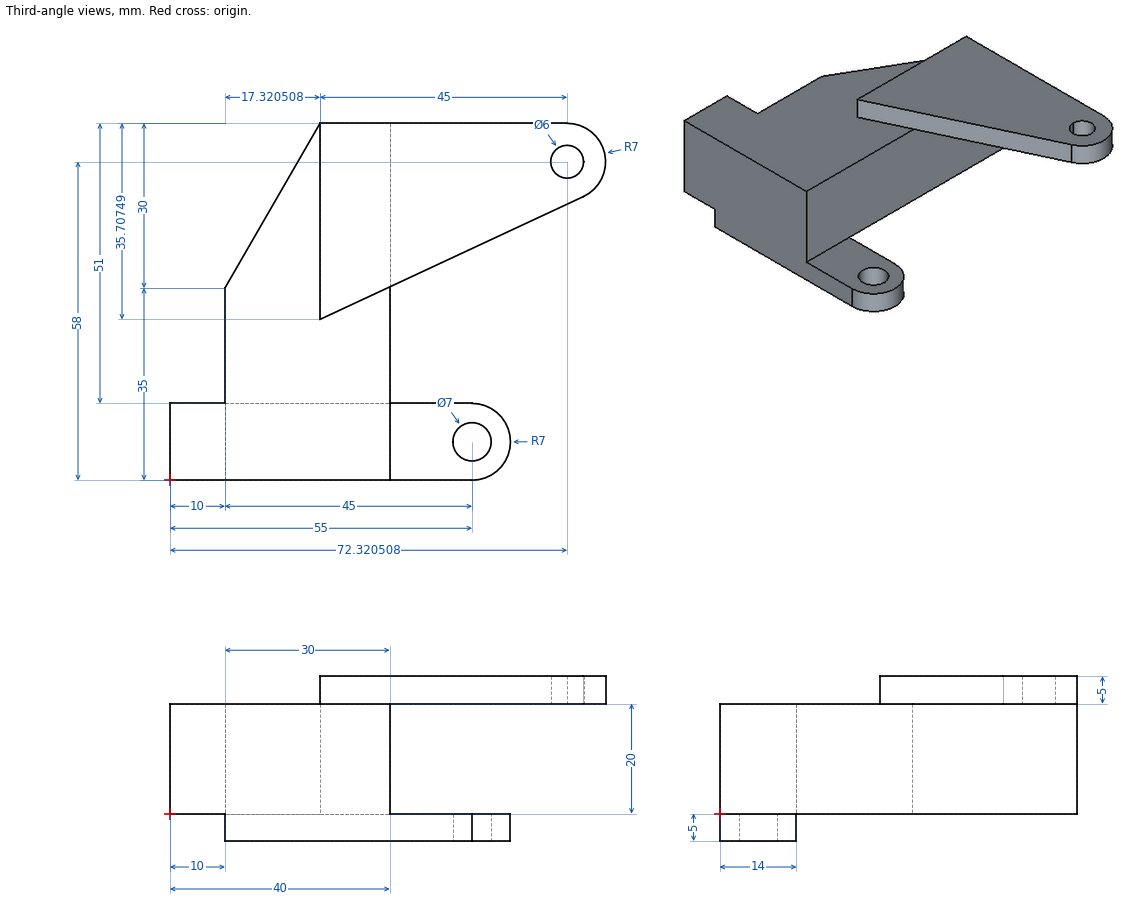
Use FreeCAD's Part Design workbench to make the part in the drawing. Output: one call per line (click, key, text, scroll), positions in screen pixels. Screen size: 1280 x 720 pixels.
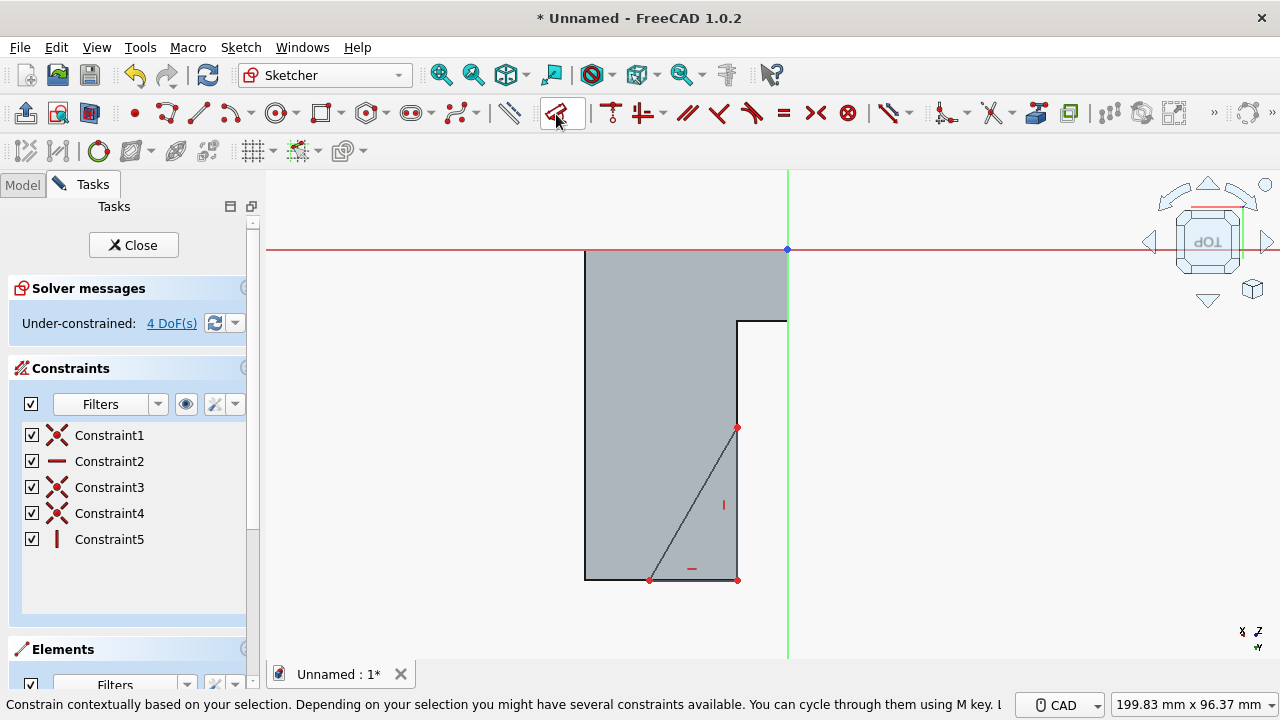
click(737, 535)
click(771, 505)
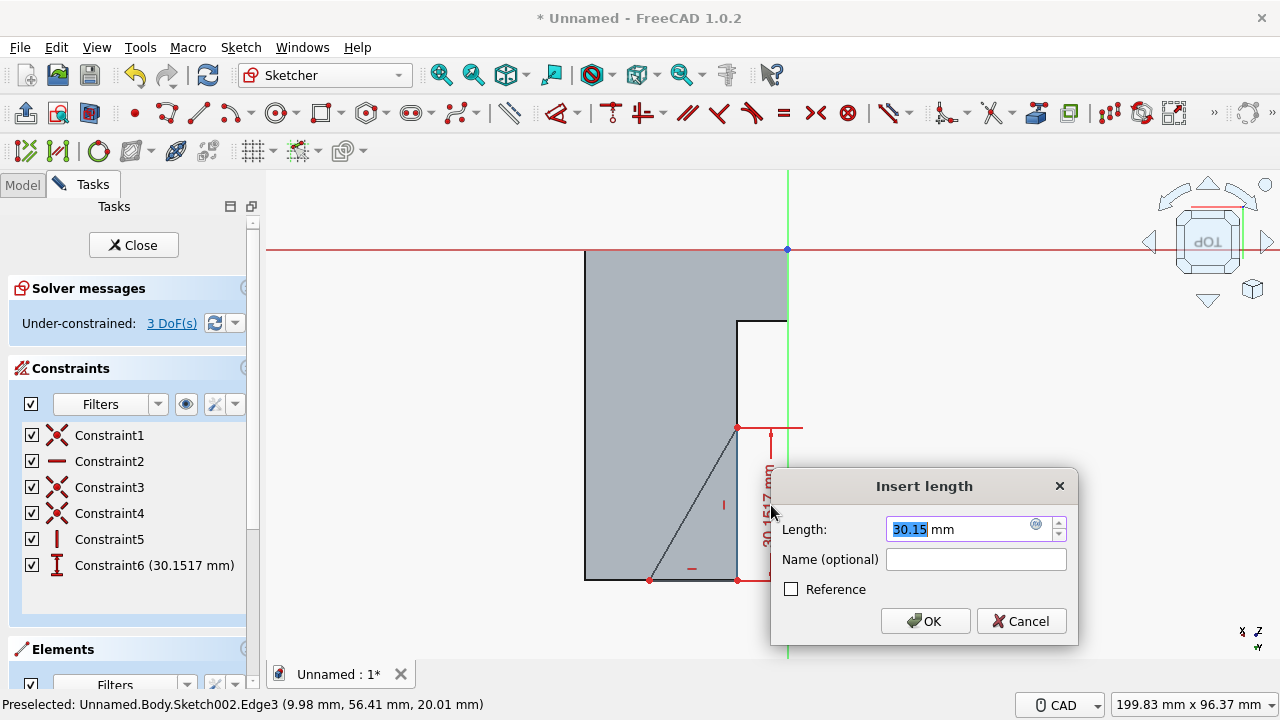
text(30)
key(Return)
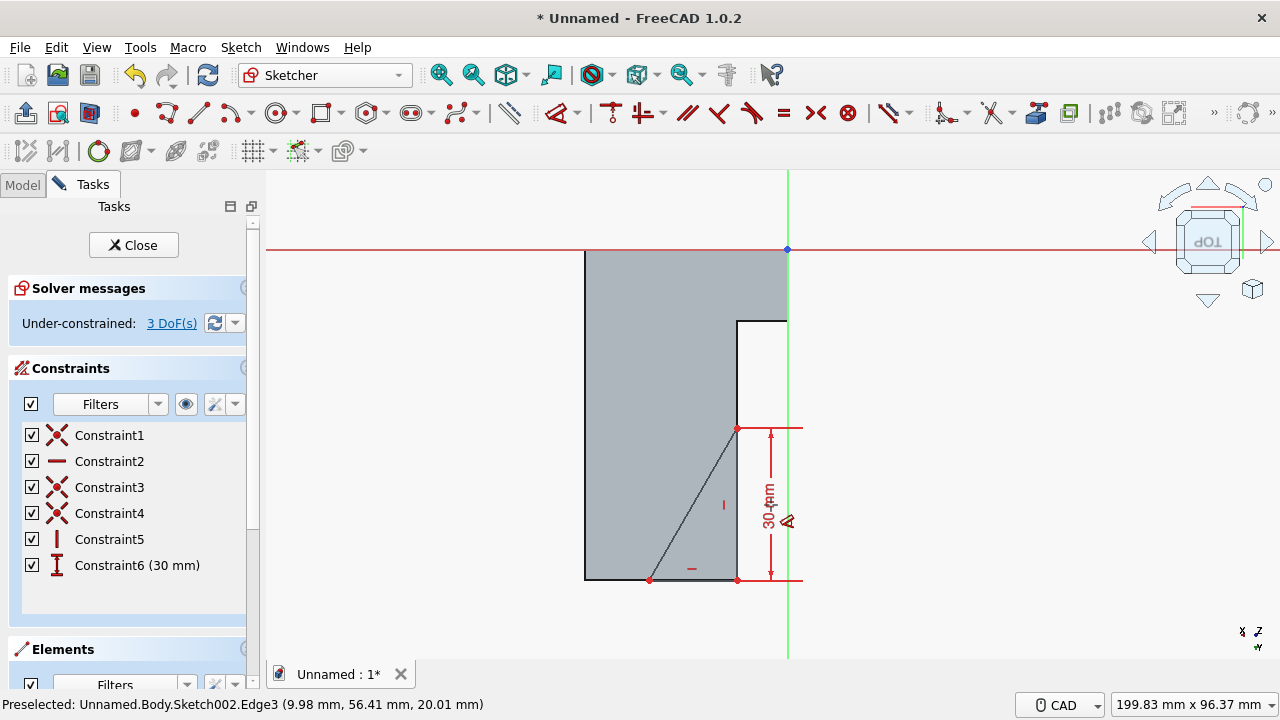
click(737, 428)
click(762, 216)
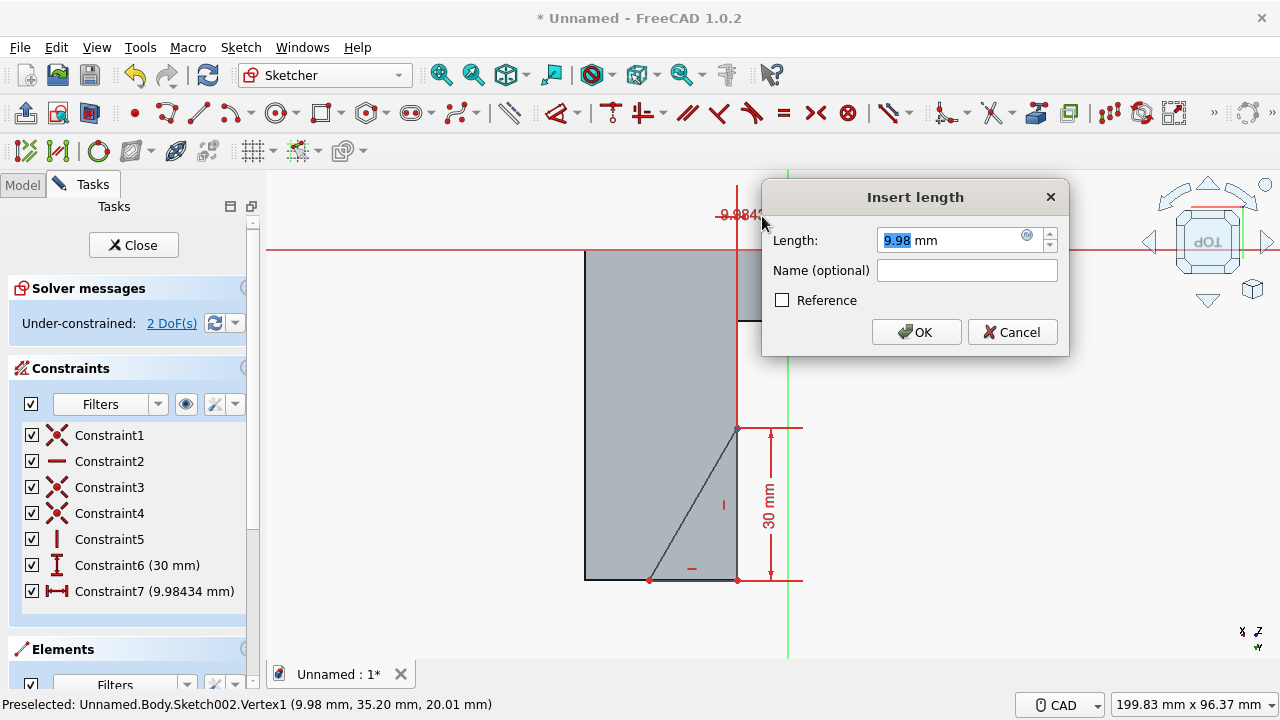
text(10)
key(Return)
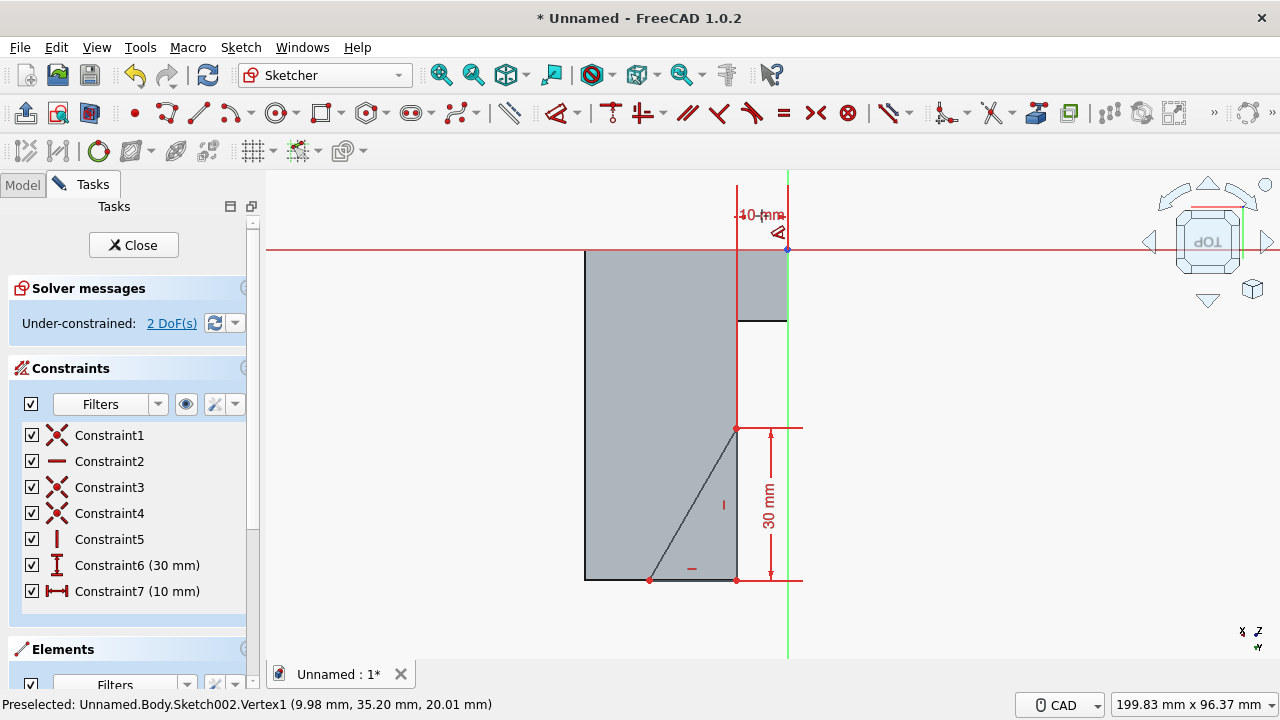
click(737, 428)
click(822, 339)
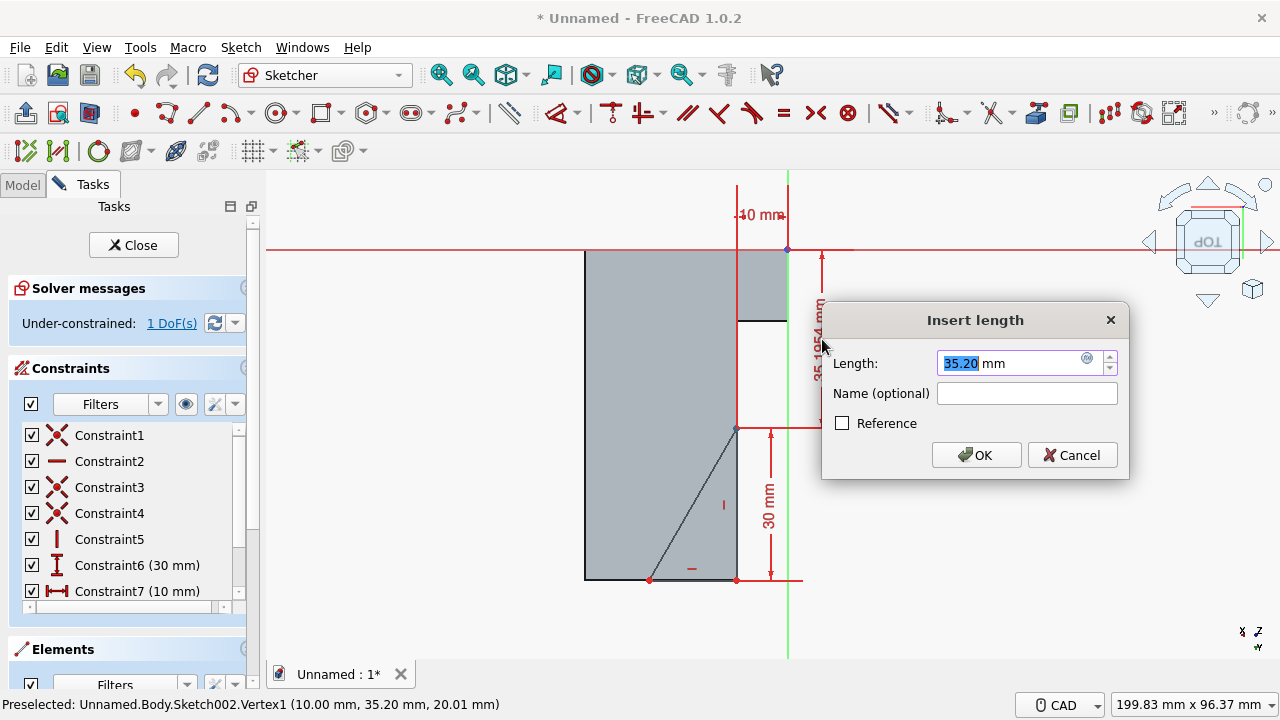
text(35)
key(Return)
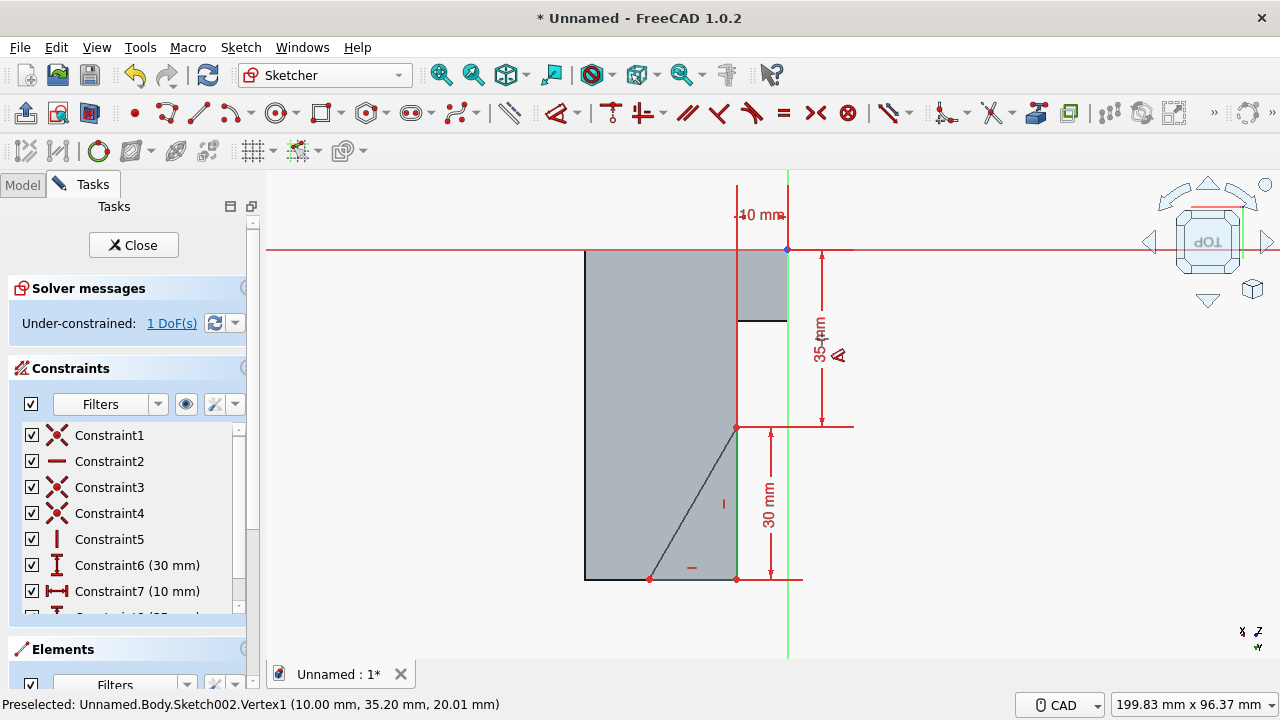
click(675, 580)
click(693, 614)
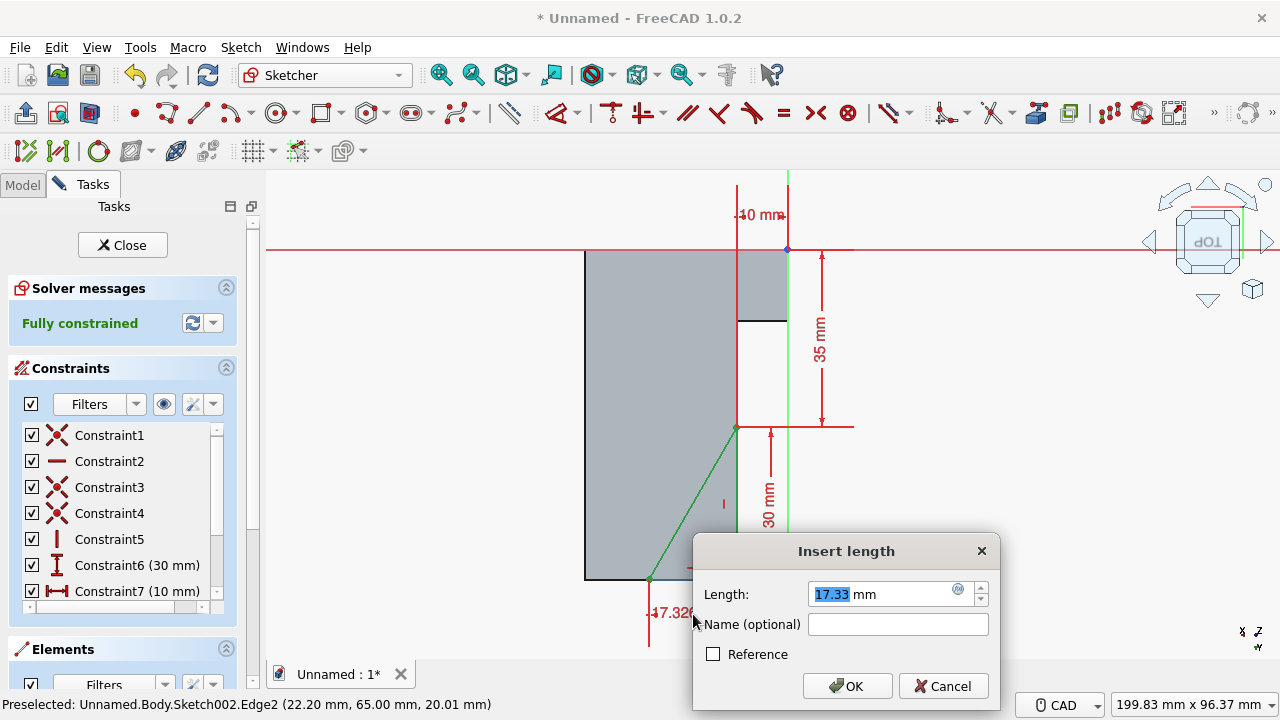
text(17.320508)
key(Return)
key(Escape)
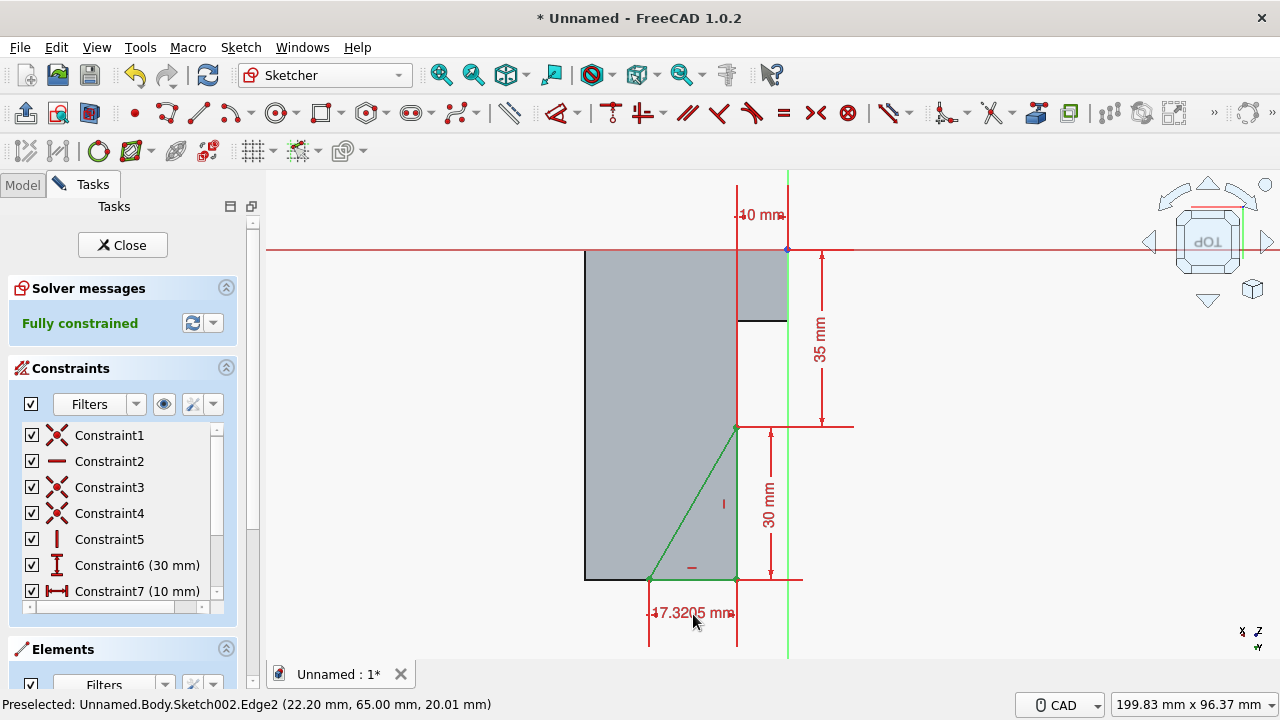
click(123, 245)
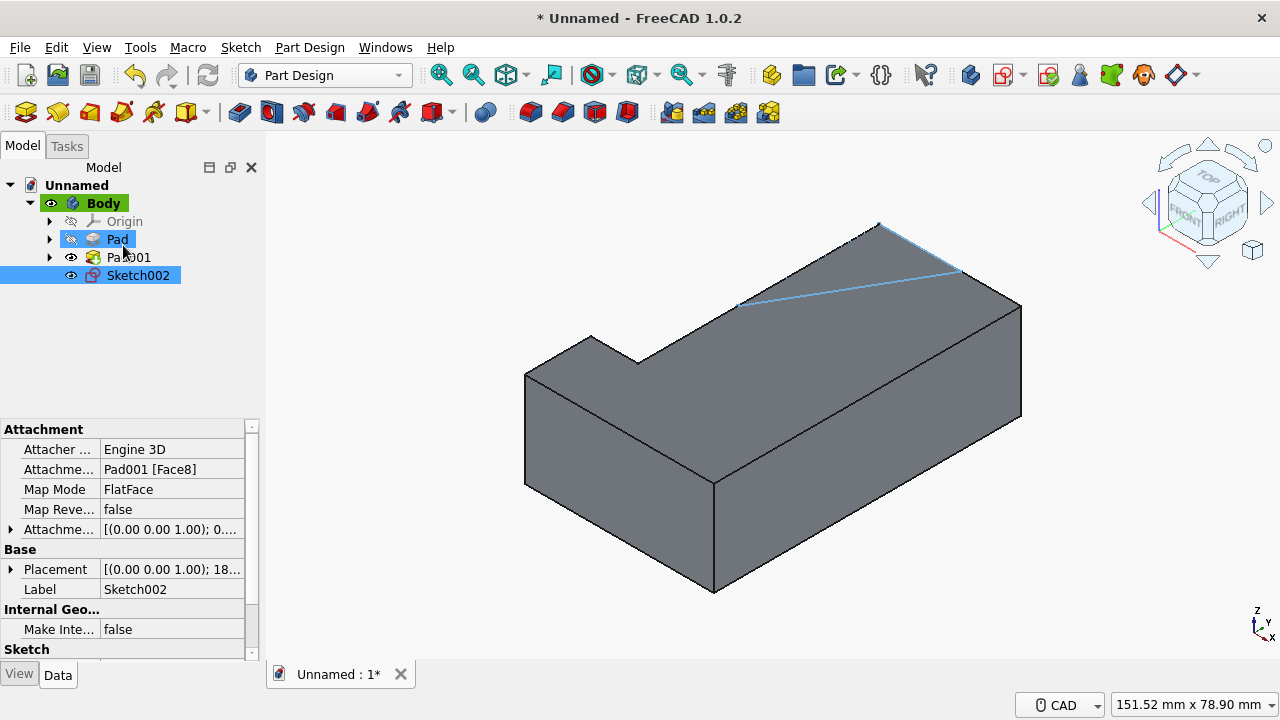
click(240, 112)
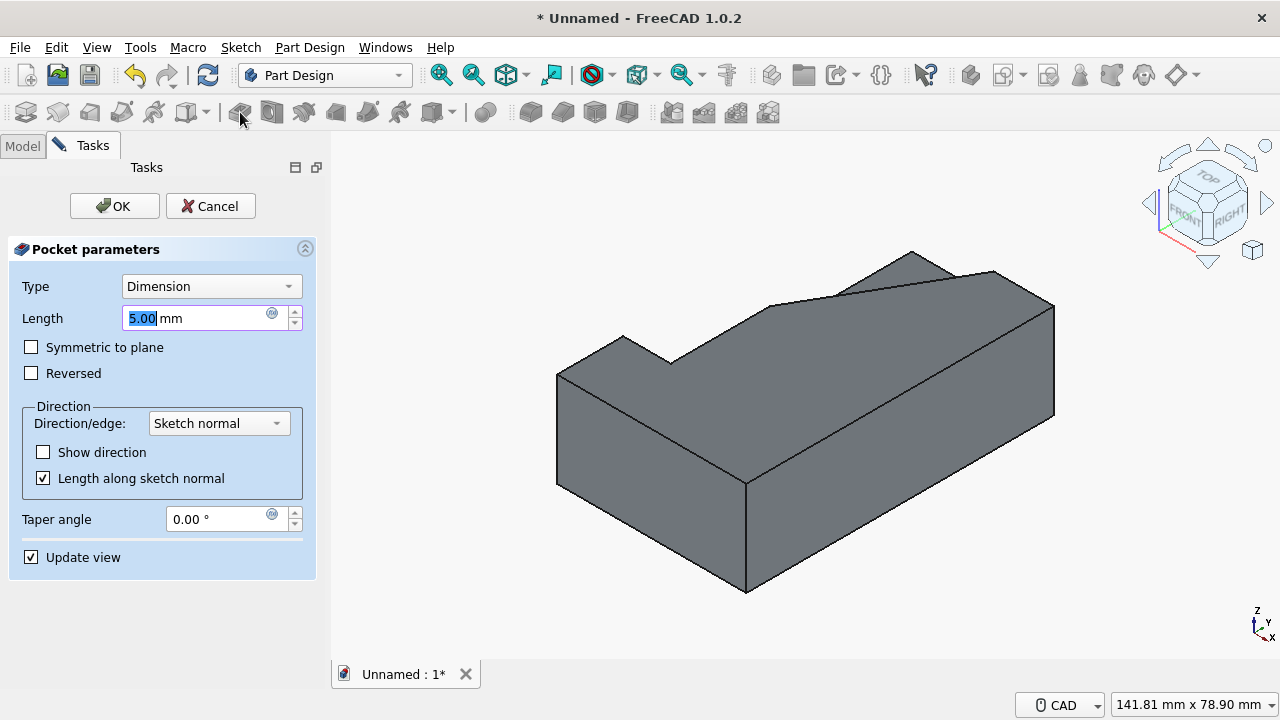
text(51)
key(Tab)